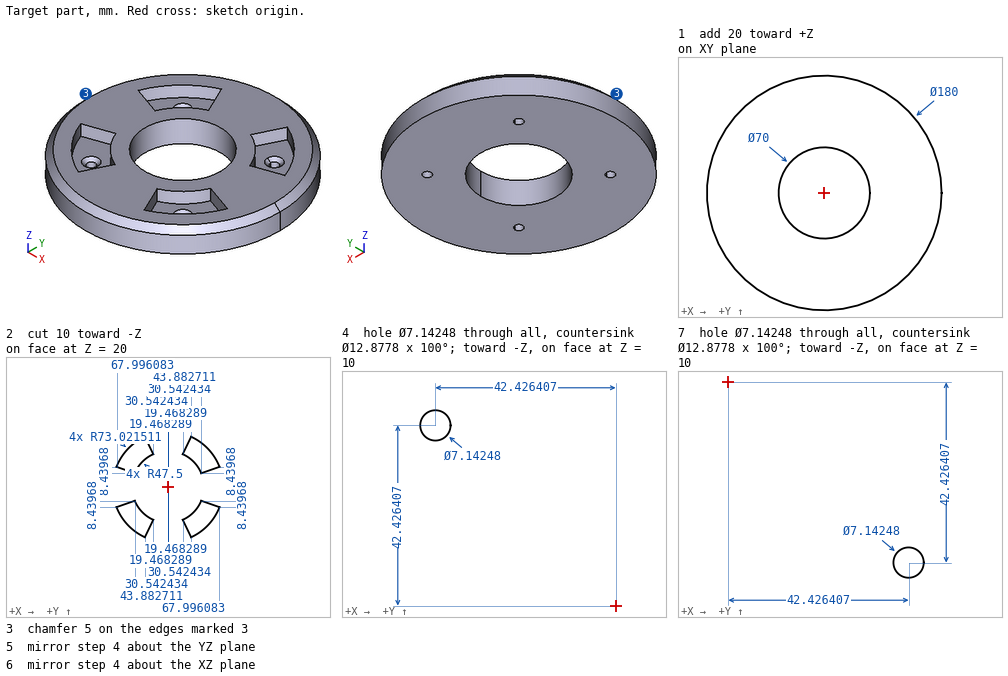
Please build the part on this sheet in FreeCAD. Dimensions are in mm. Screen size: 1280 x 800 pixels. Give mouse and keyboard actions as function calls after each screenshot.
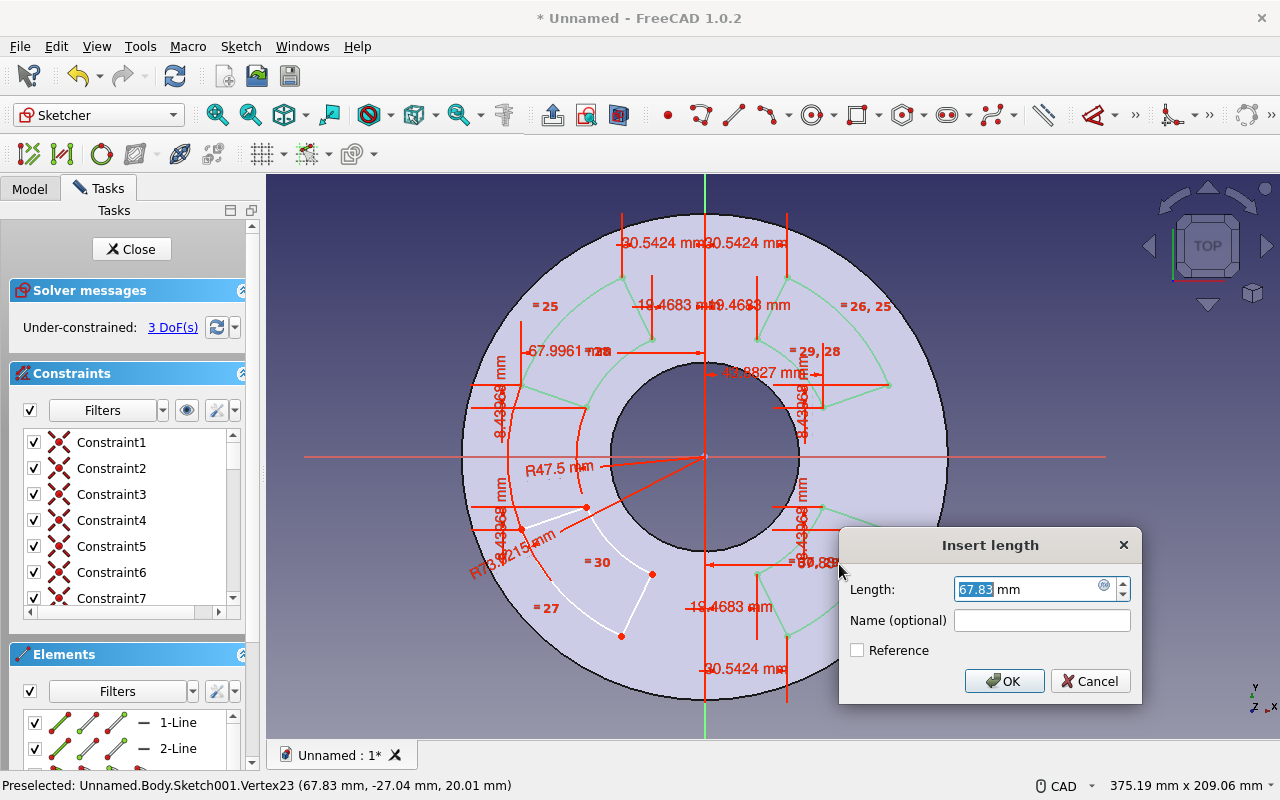
text(67.996083)
key(Return)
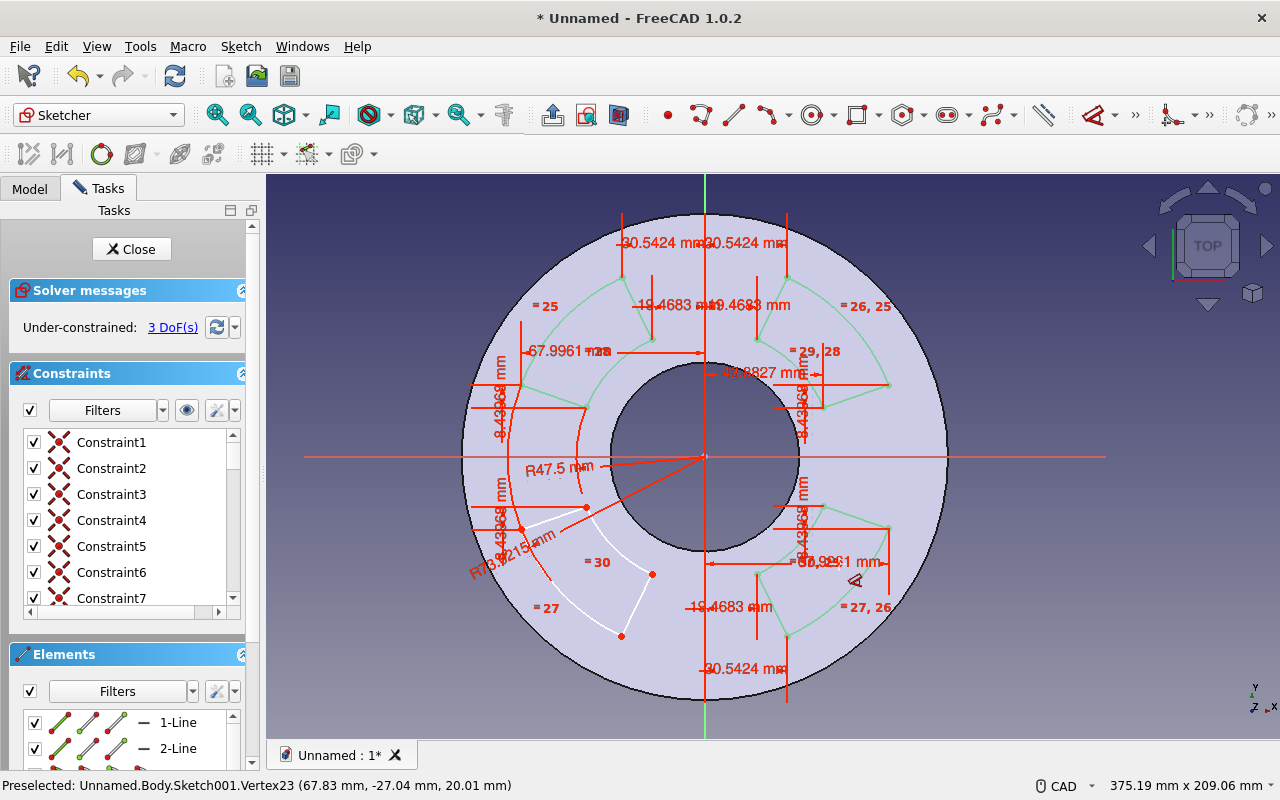
click(587, 507)
click(646, 541)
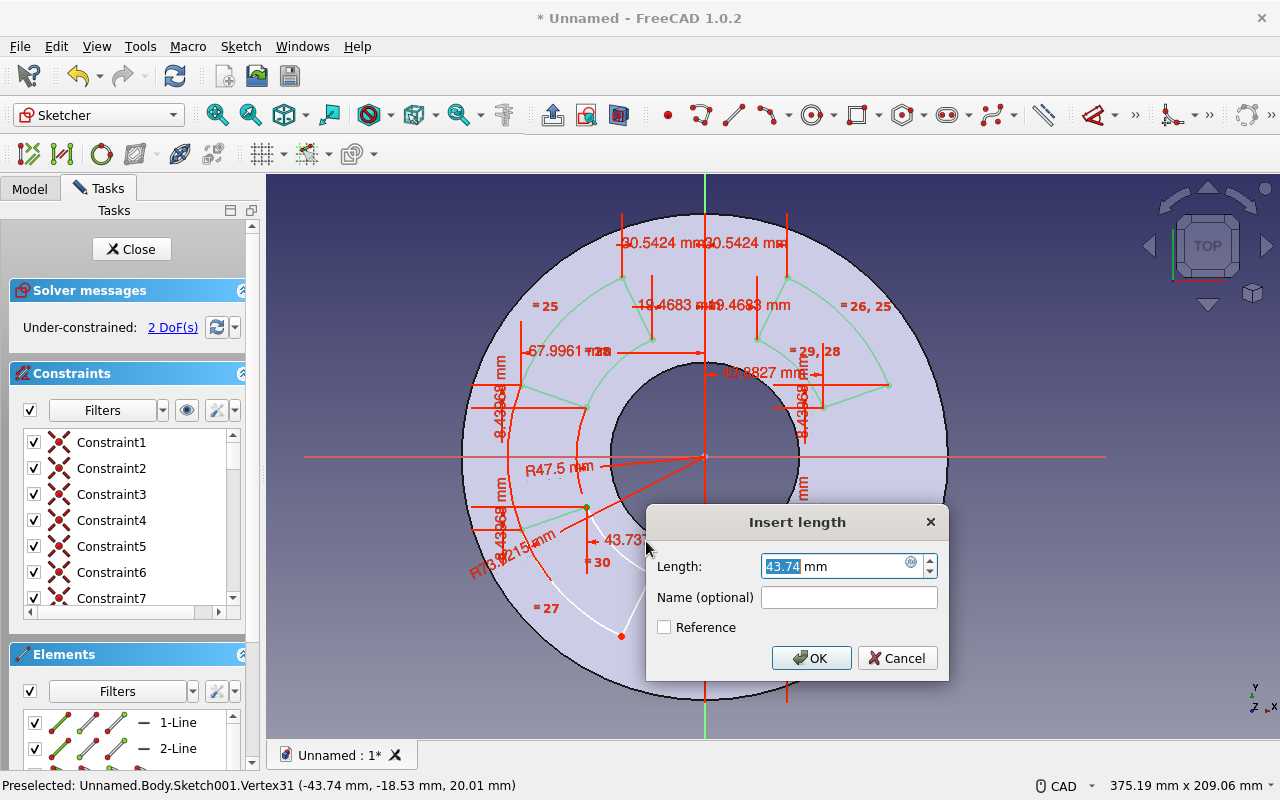
text(43.882711)
key(Return)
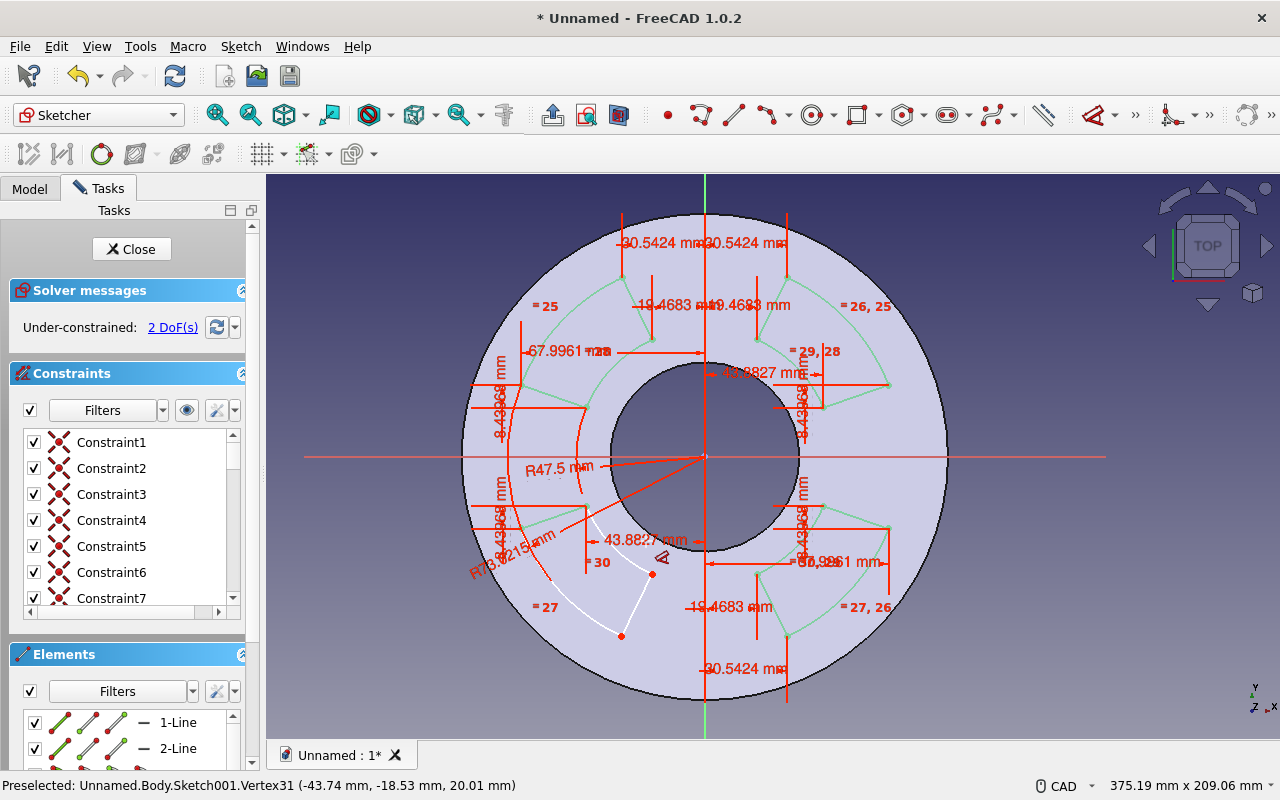
click(622, 636)
click(663, 670)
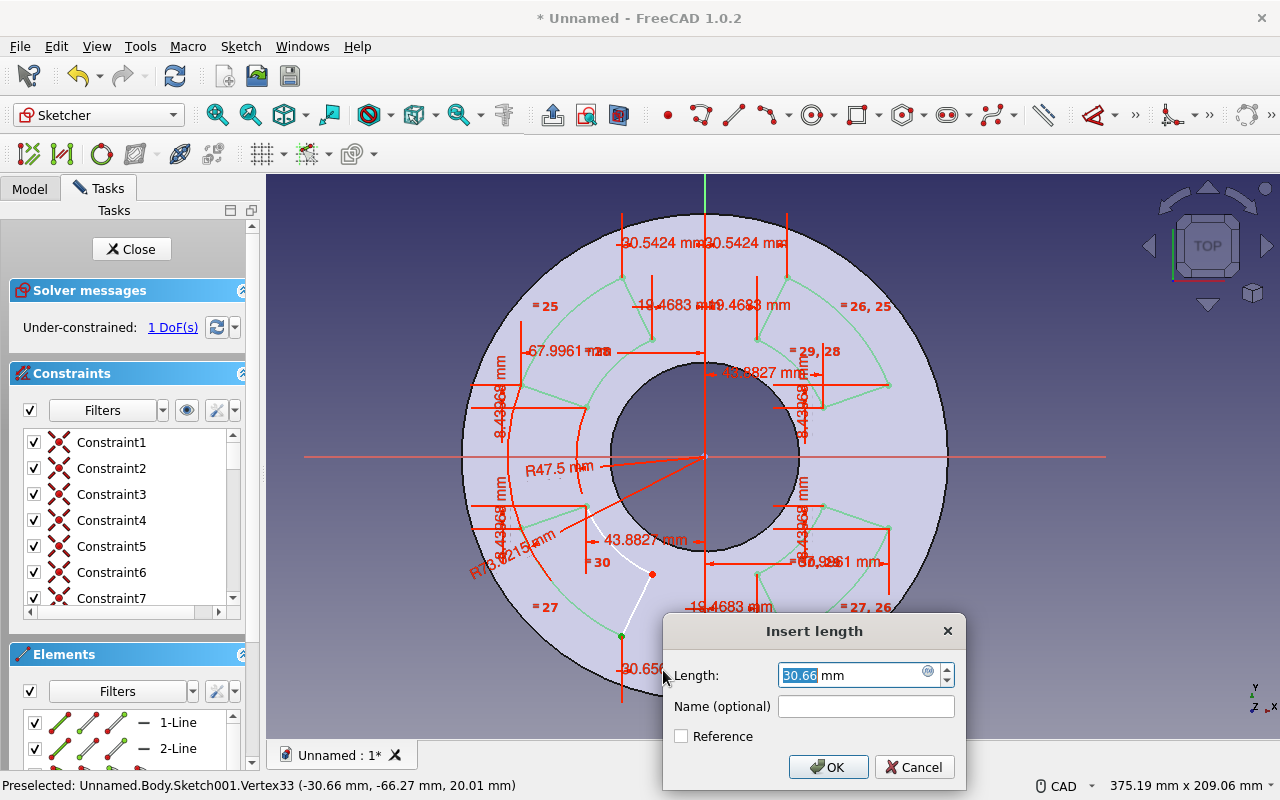
text(30.542434)
key(Return)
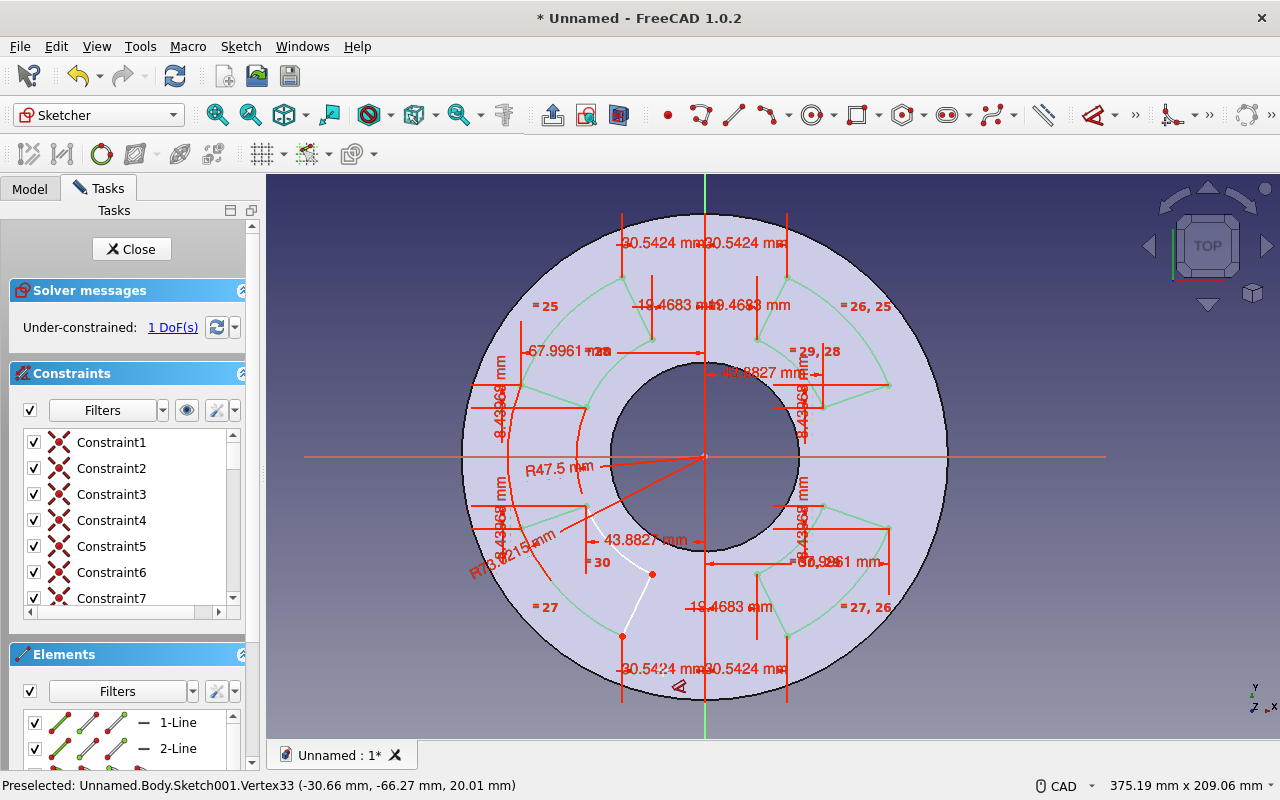
click(652, 574)
click(660, 608)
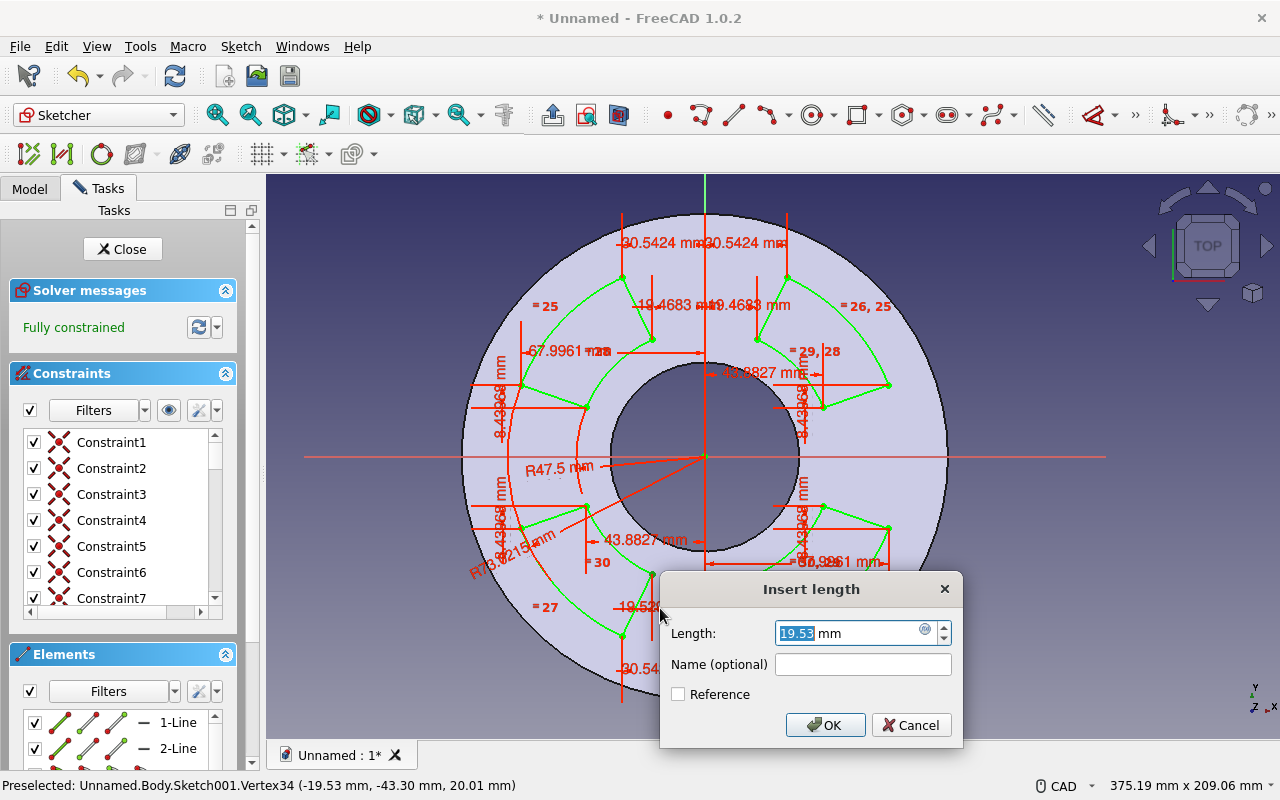
text(19.468289)
key(Return)
key(Escape)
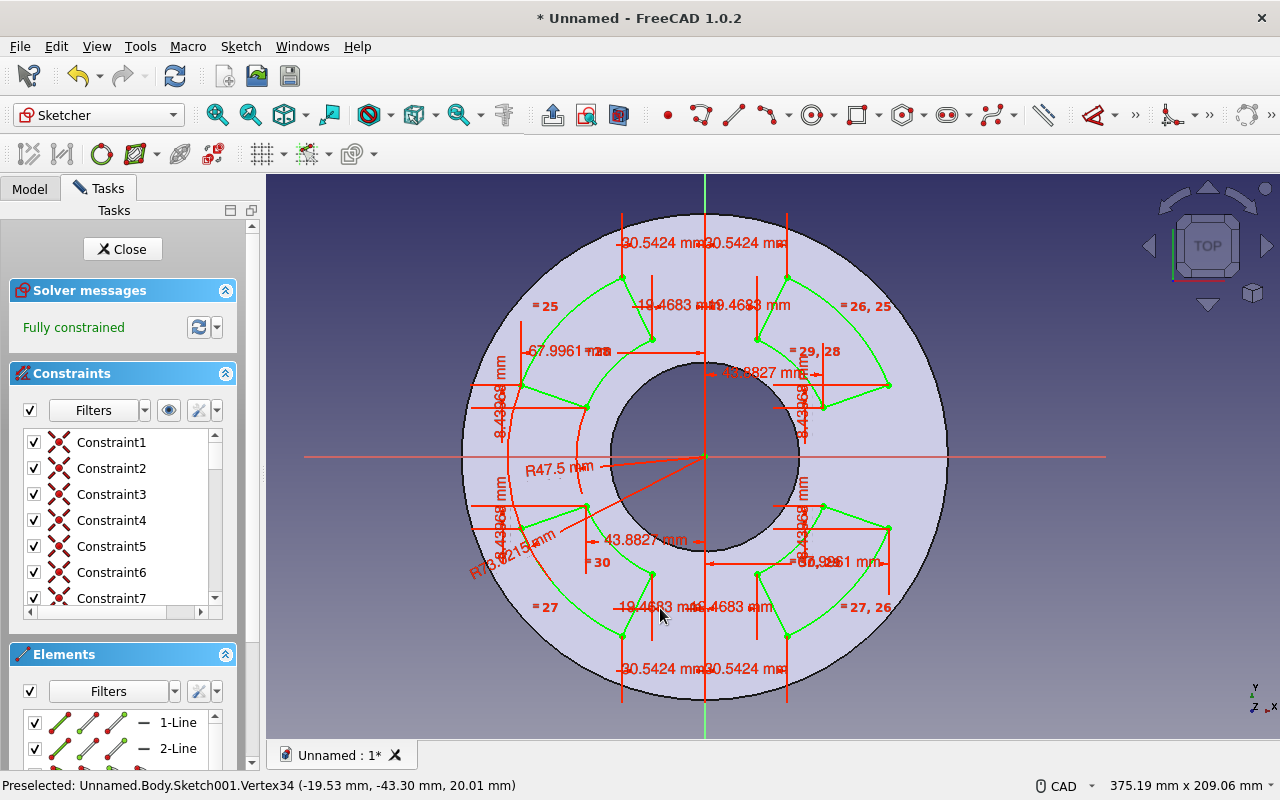
click(123, 249)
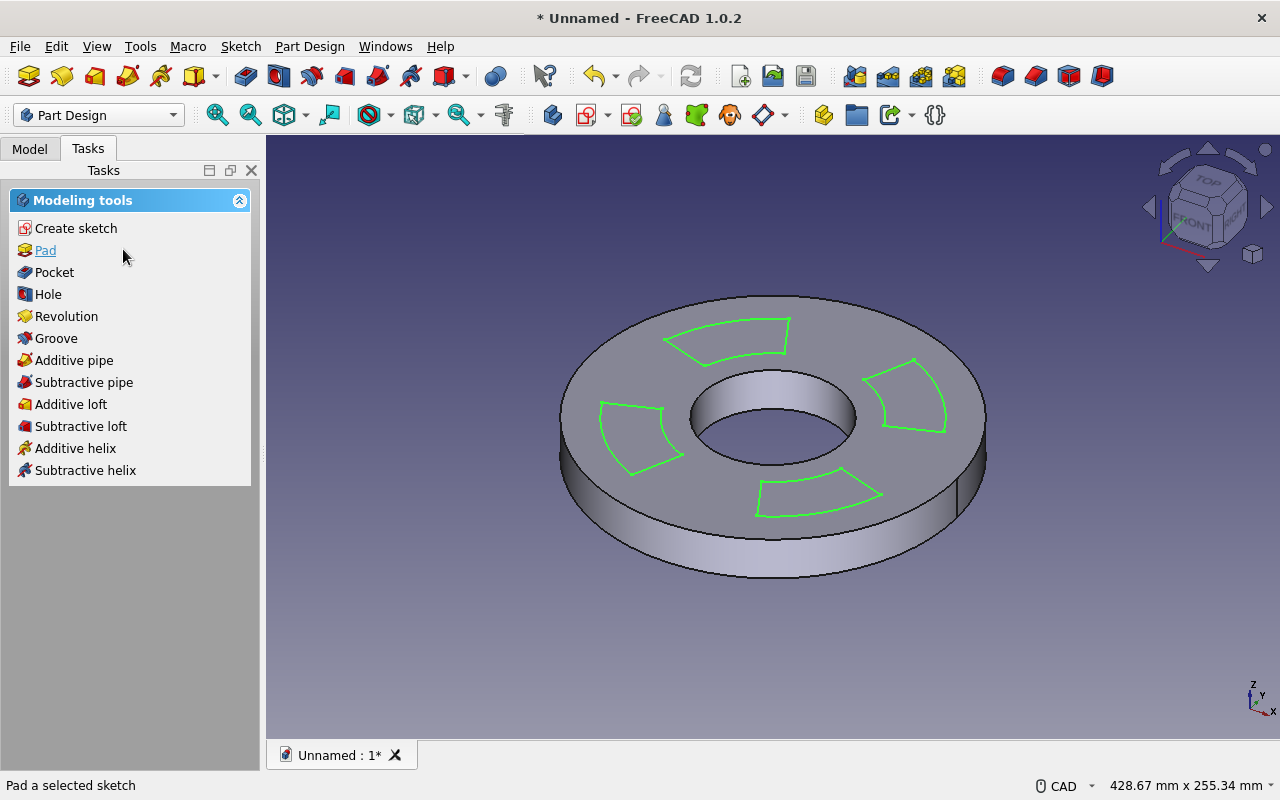
click(246, 76)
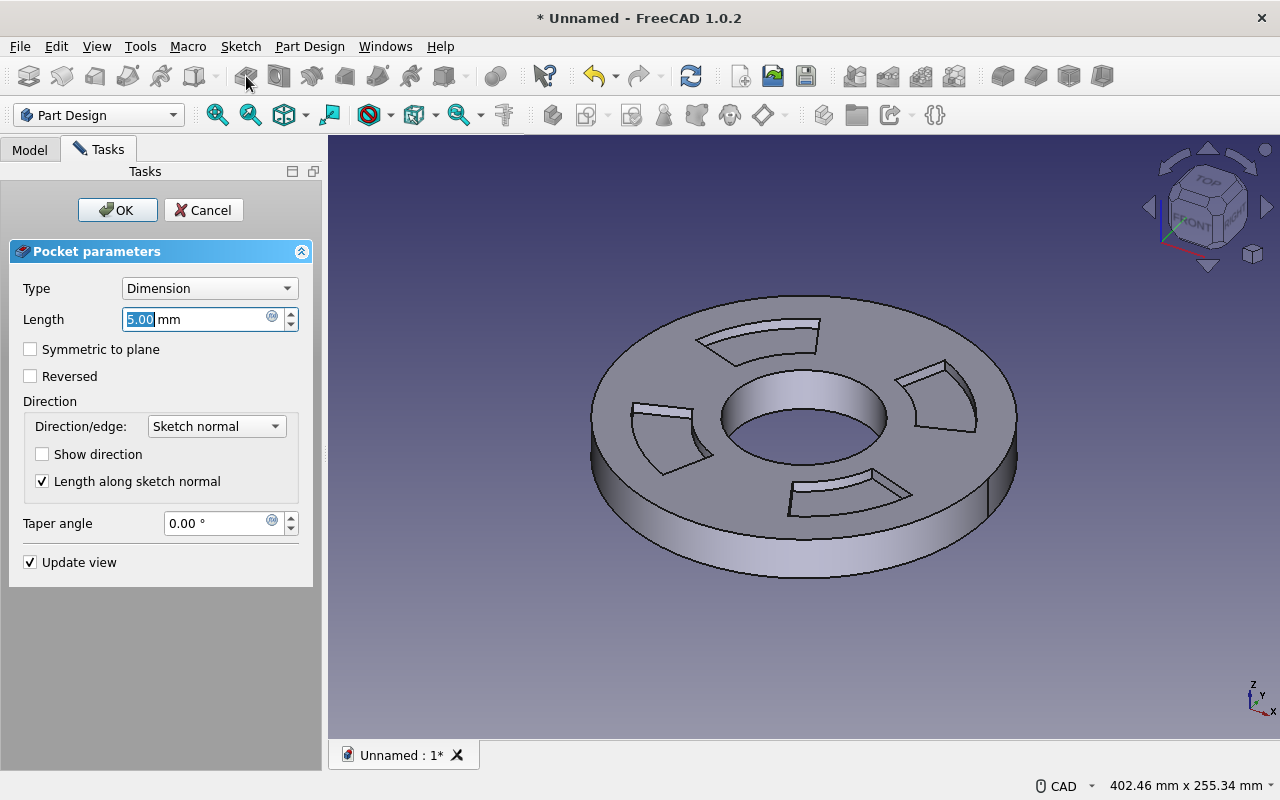
text(10)
key(Tab)